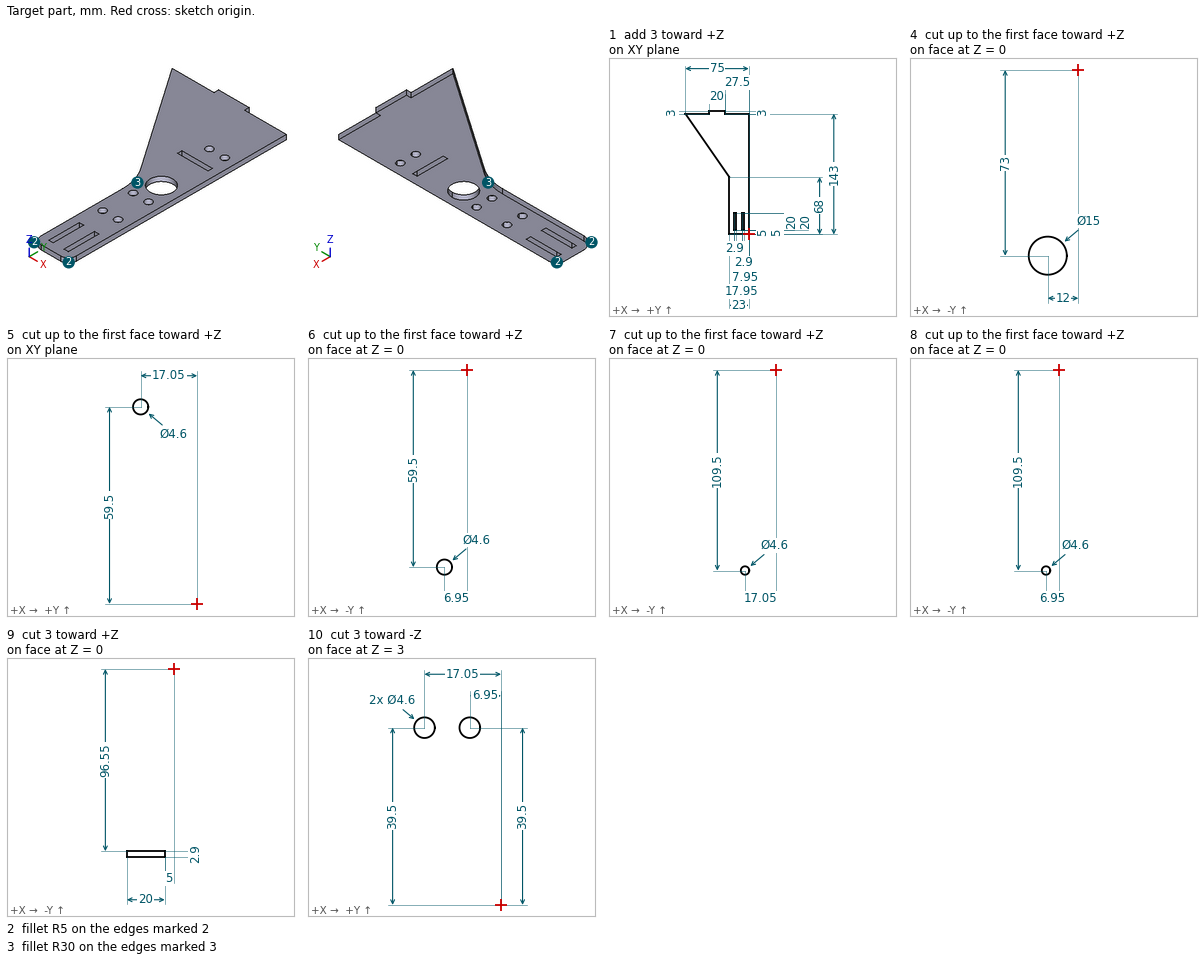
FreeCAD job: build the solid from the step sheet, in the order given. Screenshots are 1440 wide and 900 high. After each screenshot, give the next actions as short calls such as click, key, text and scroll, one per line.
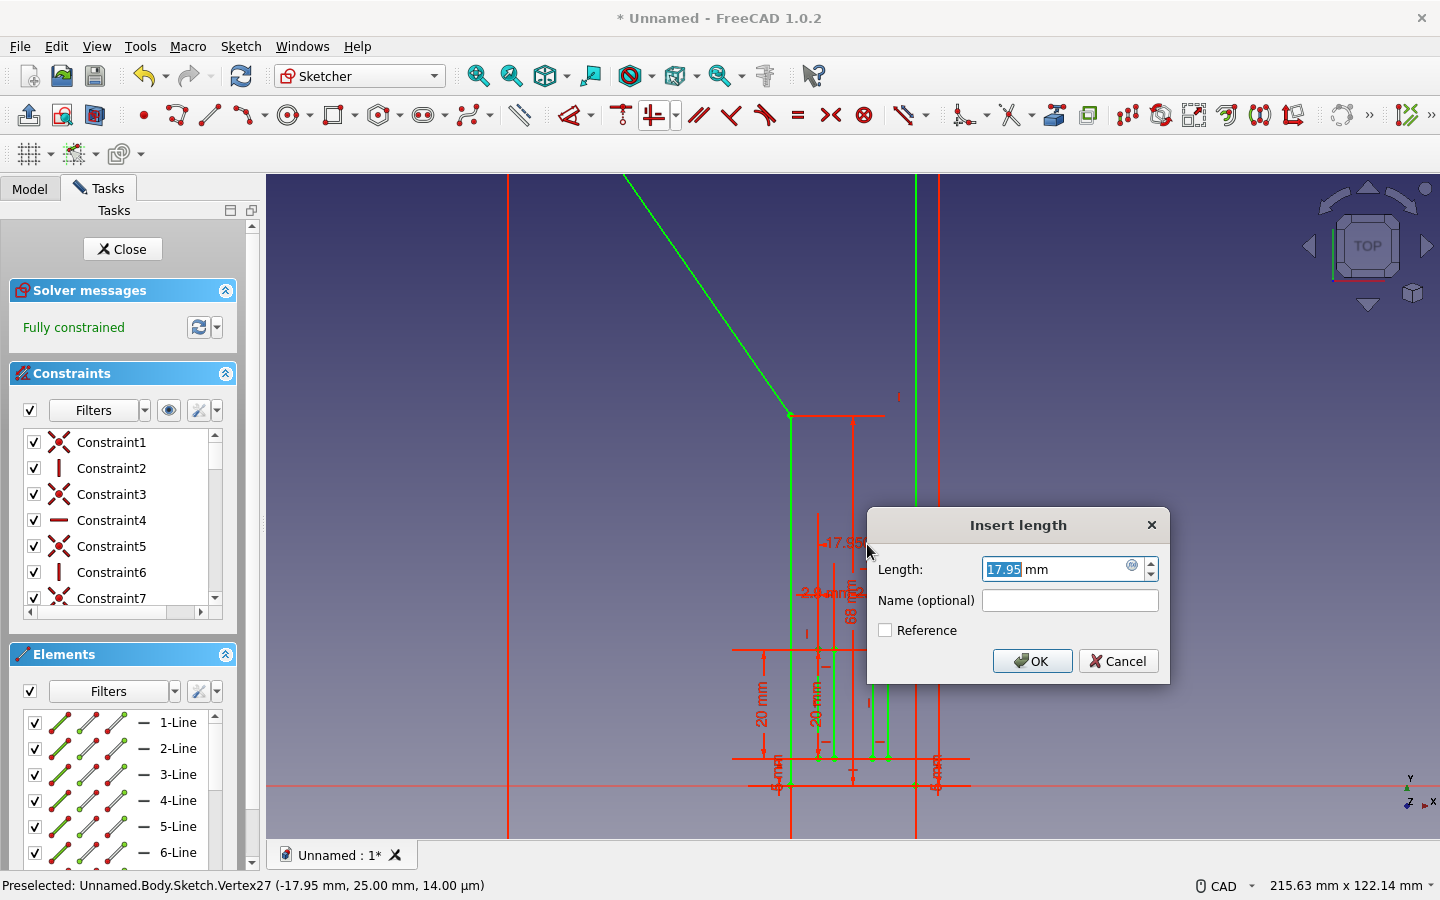
text(17.95)
key(Return)
key(Escape)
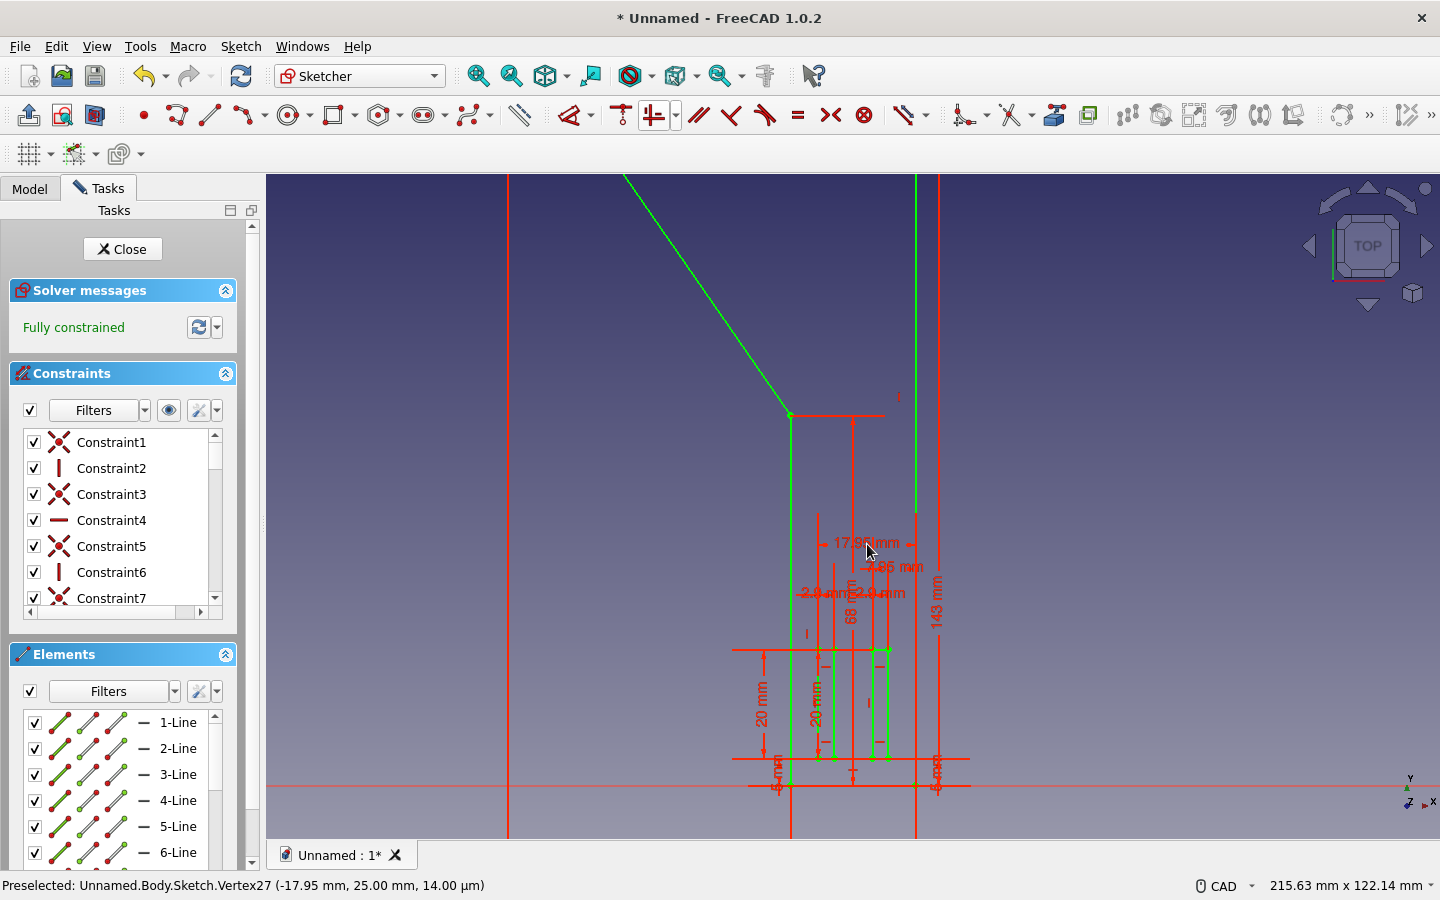
click(123, 249)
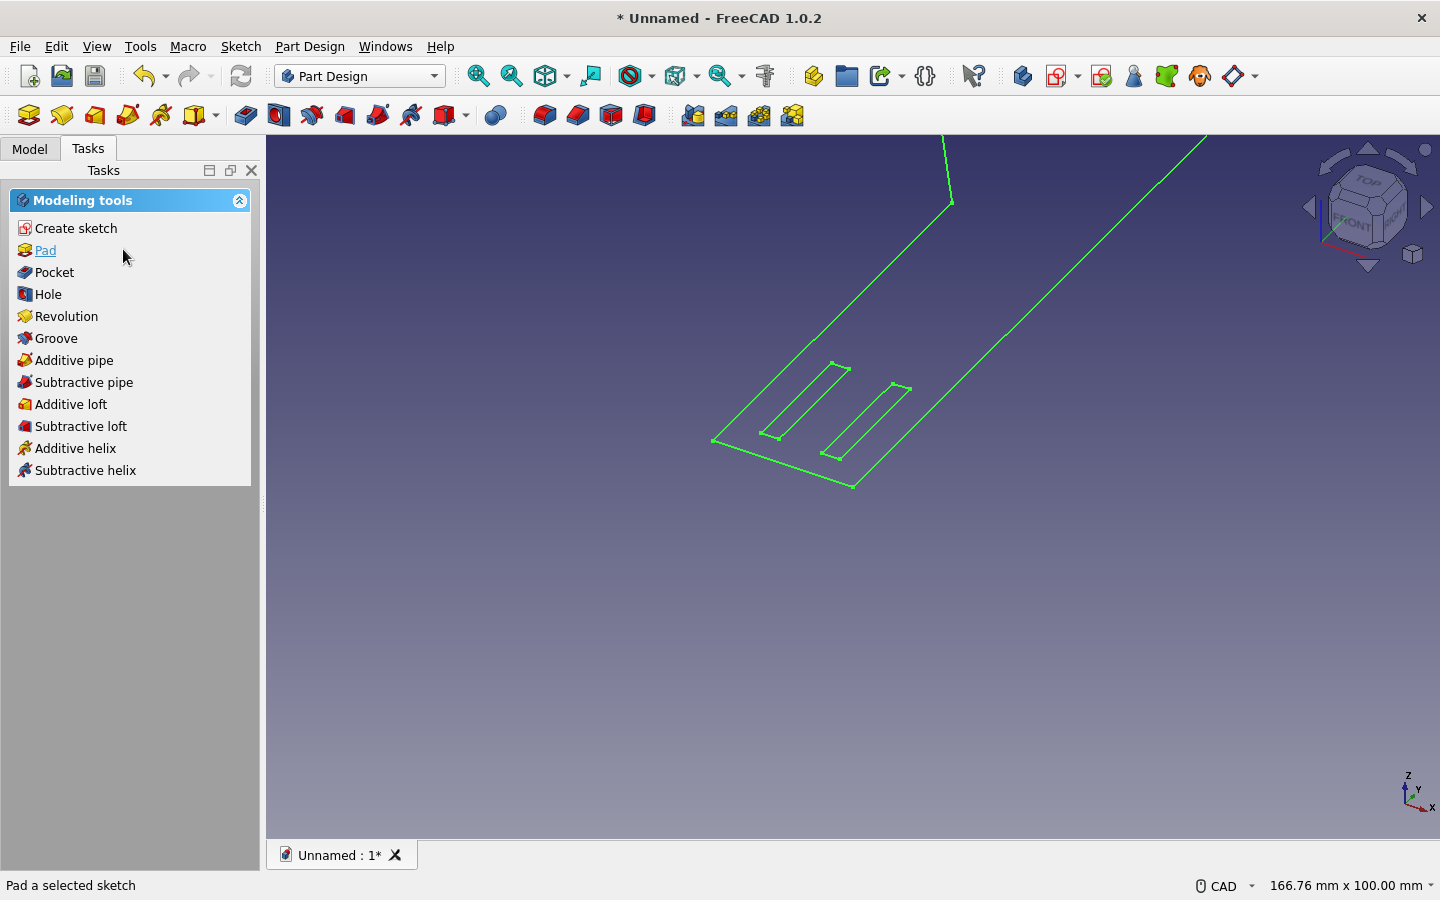
click(29, 116)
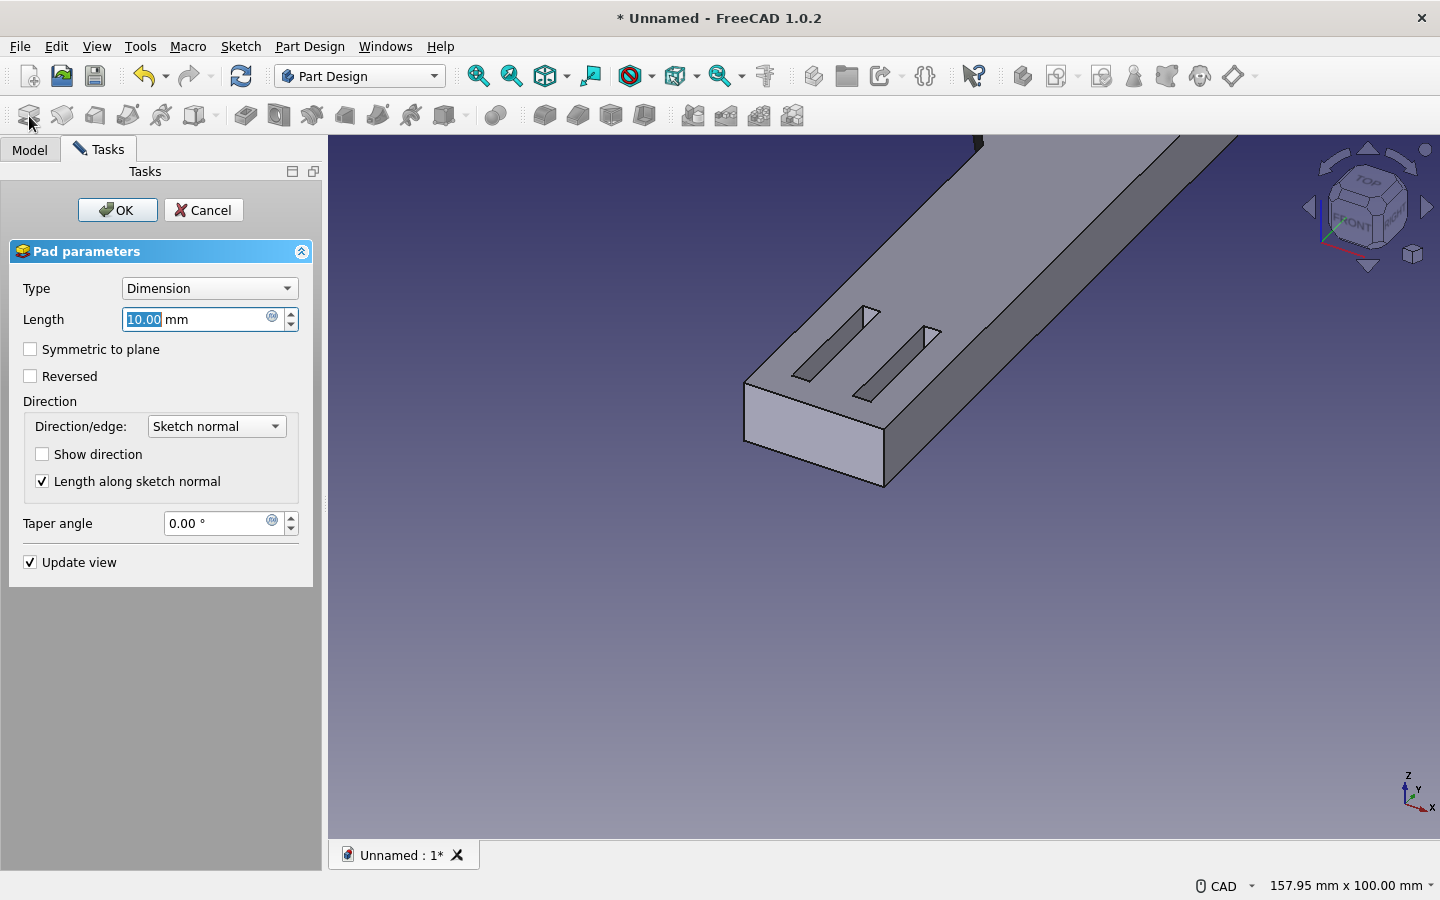
text(3)
key(Tab)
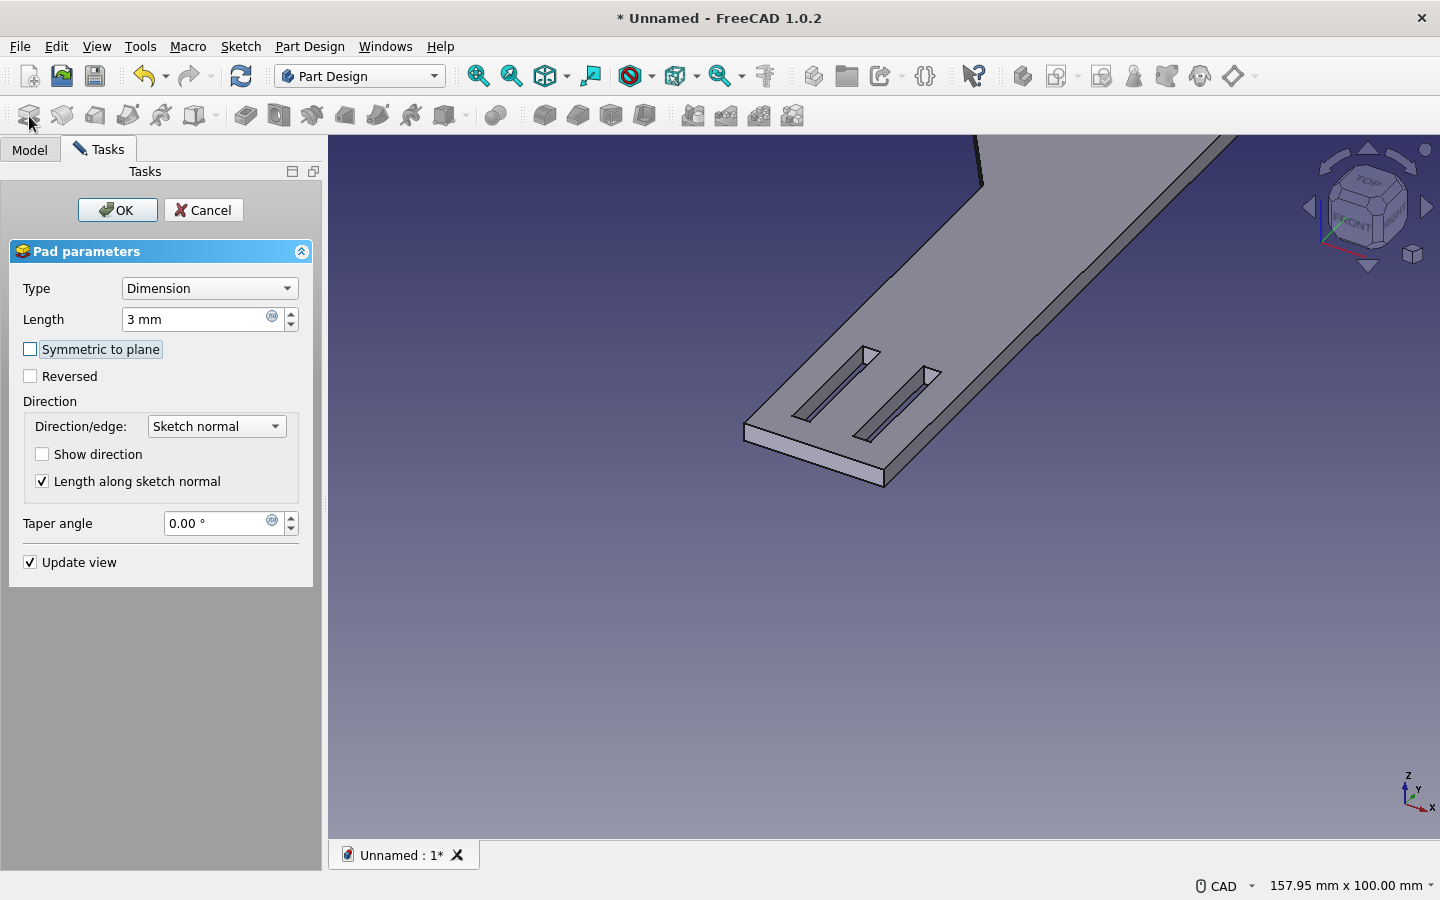
click(118, 210)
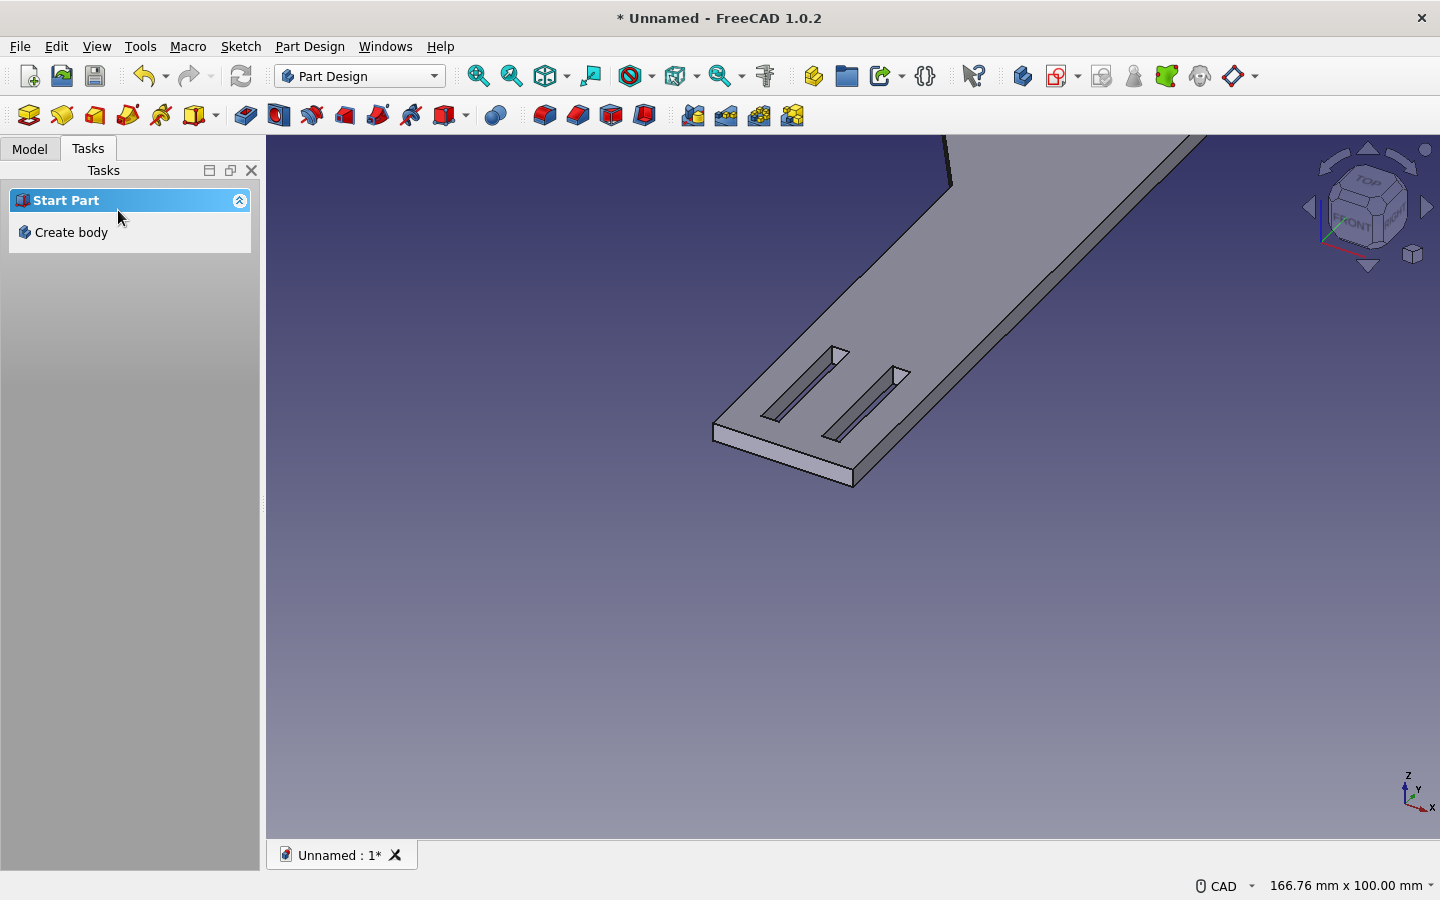
key(v)
key(f)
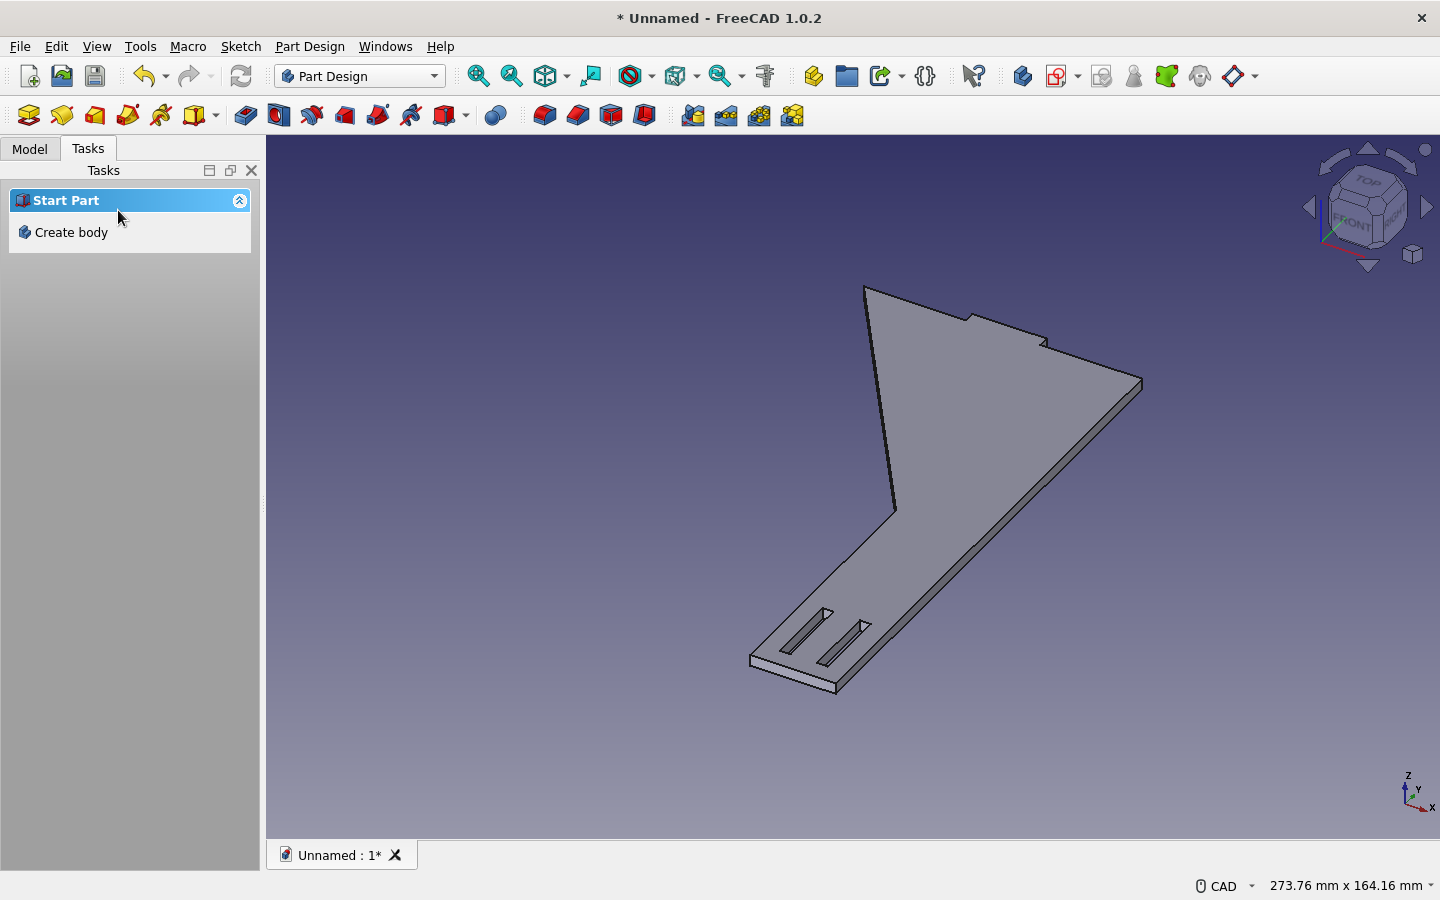
click(836, 689)